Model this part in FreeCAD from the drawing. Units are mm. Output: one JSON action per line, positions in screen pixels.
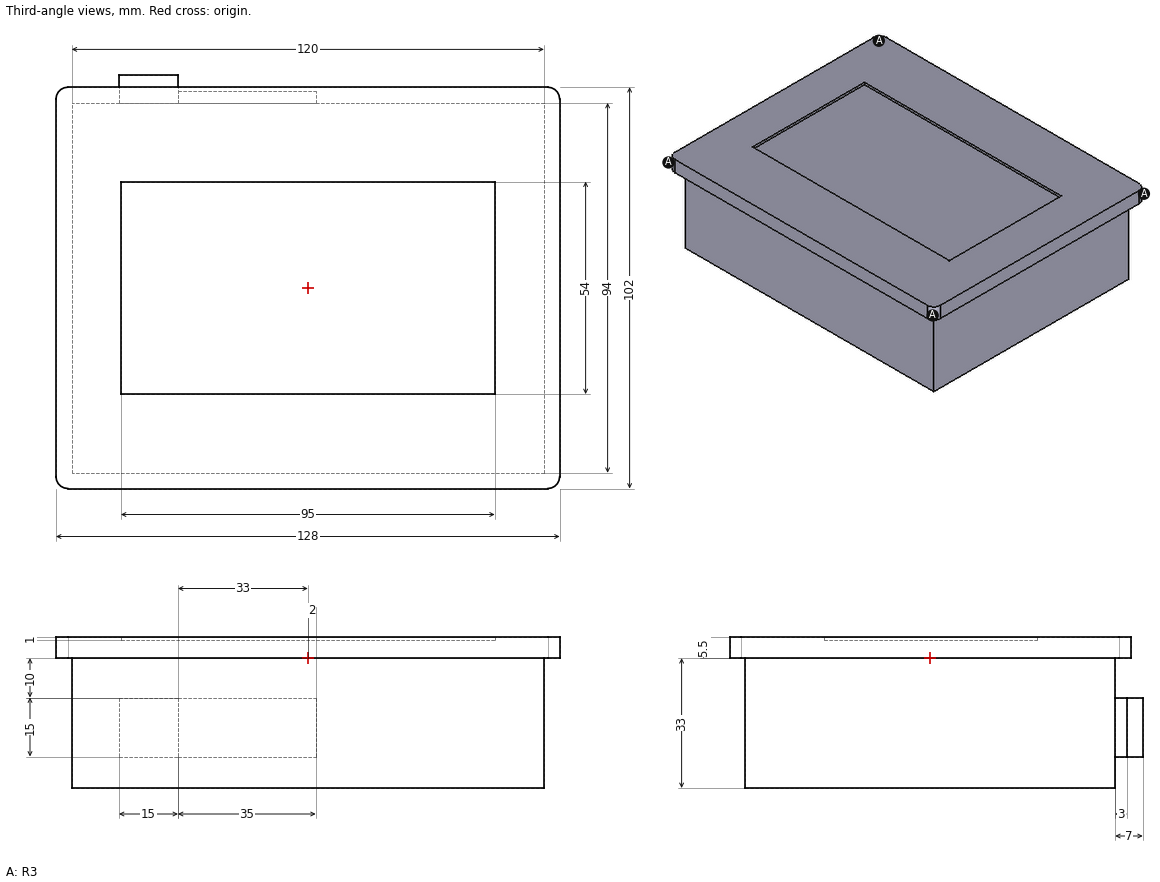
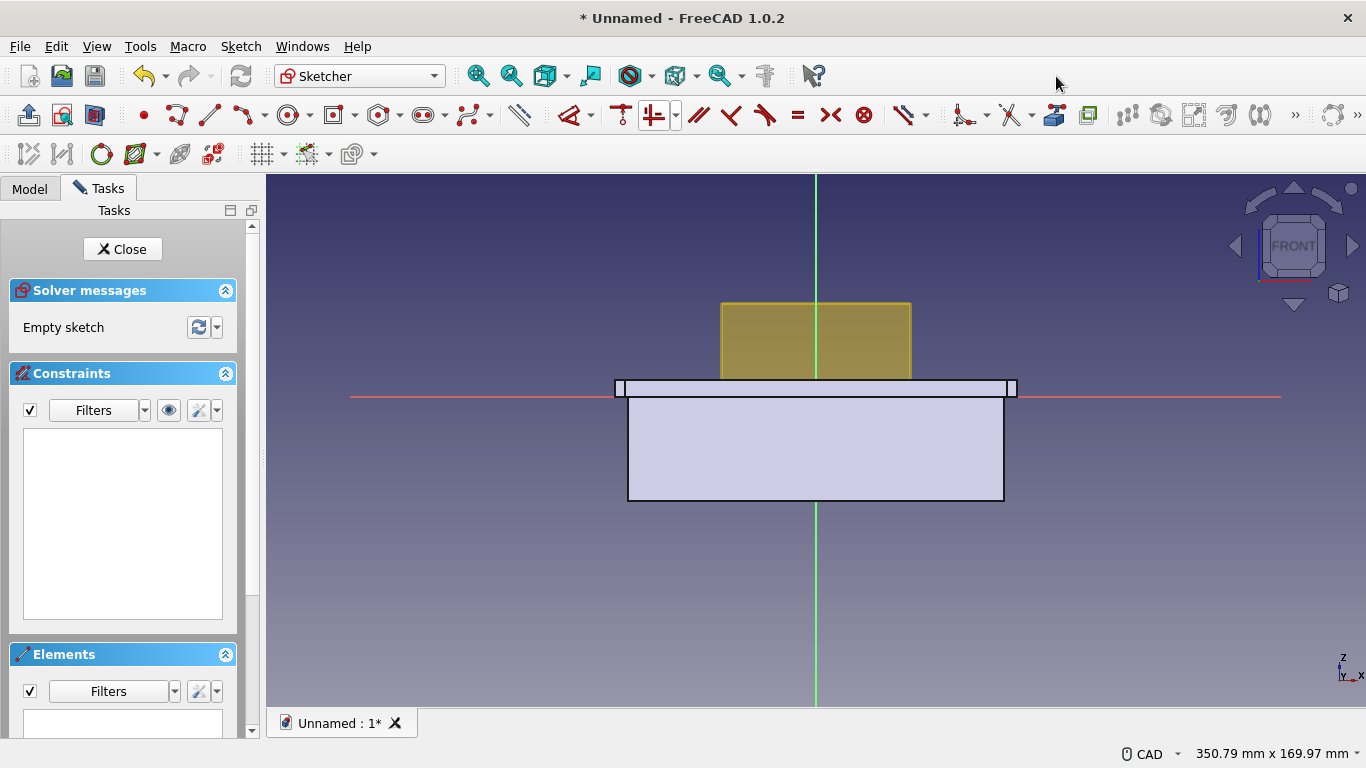
{"action": "scroll", "coordinate": [774, 435], "scroll_direction": "up", "scroll_amount": 7}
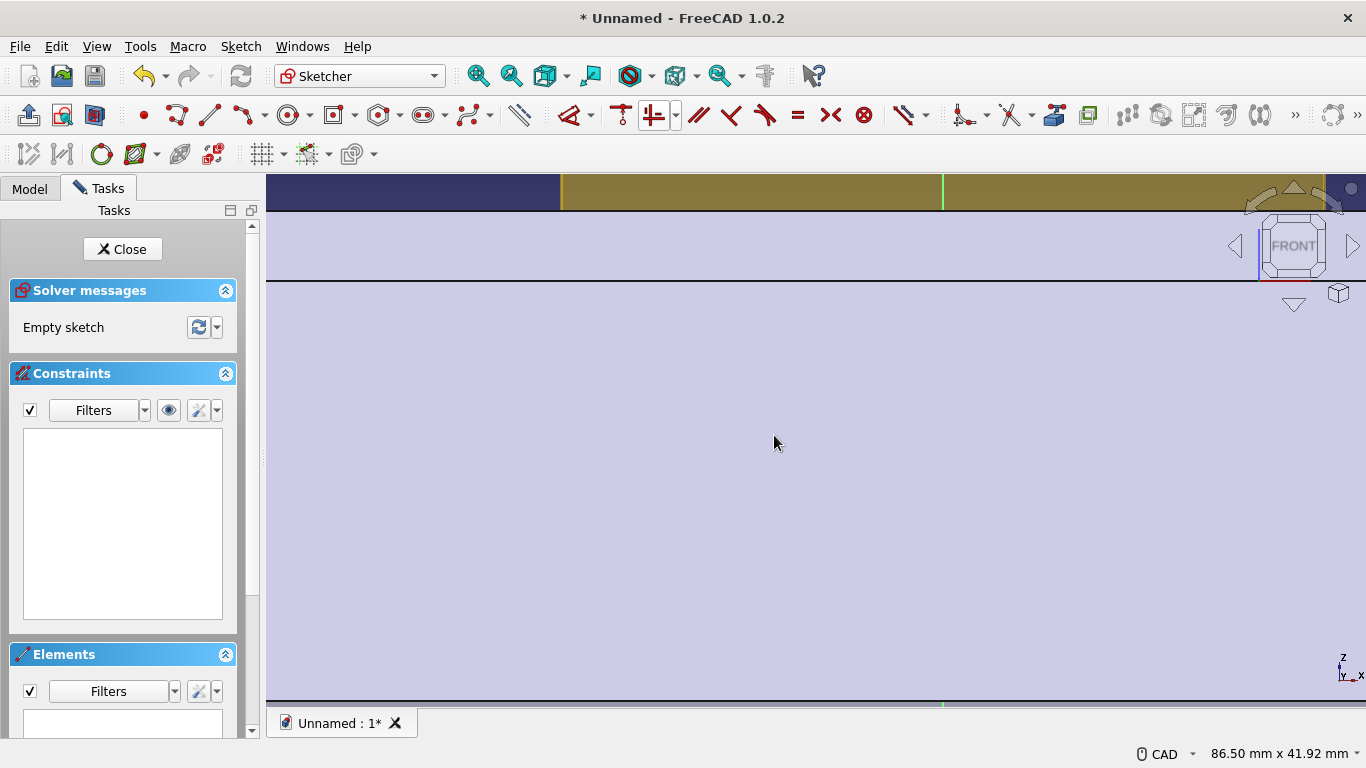
{"action": "key", "text": "g r"}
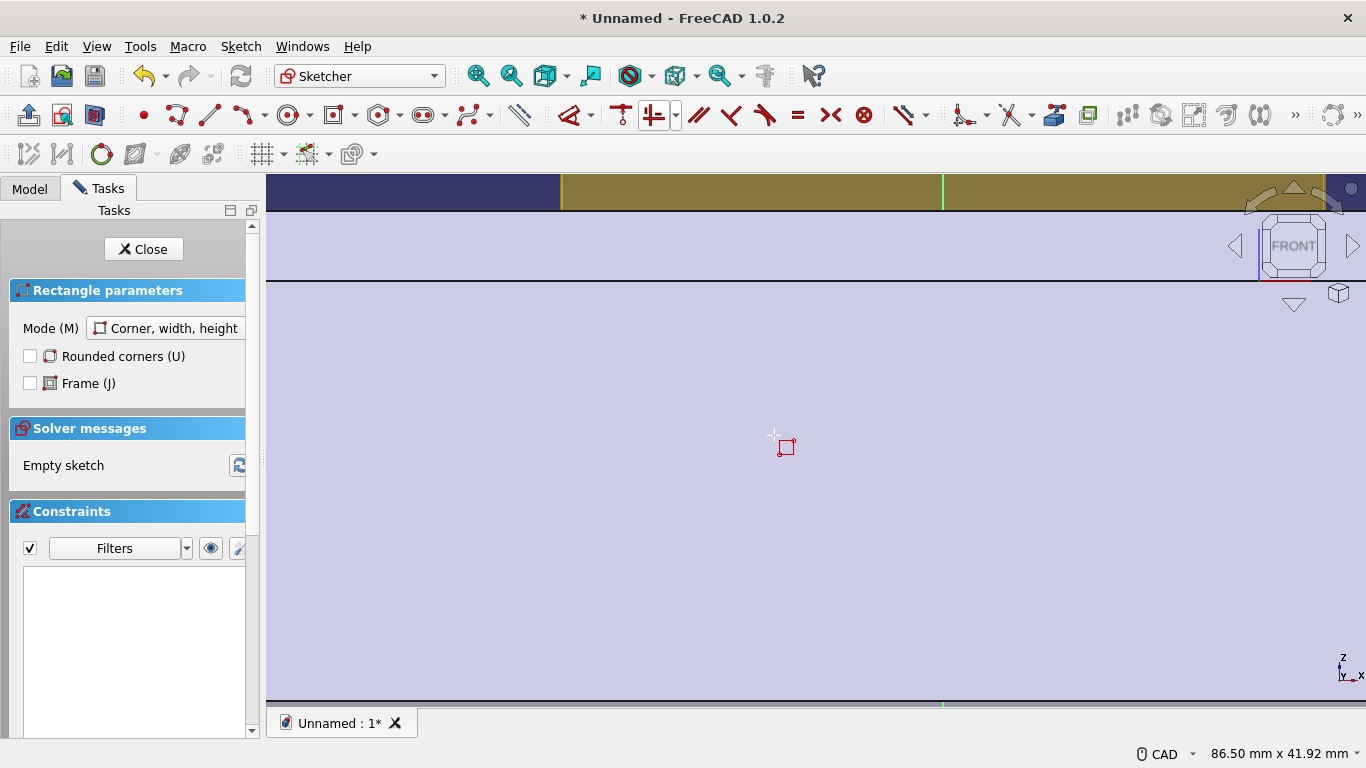
{"action": "left_click", "coordinate": [523, 408]}
{"action": "mouse_move", "coordinate": [968, 599]}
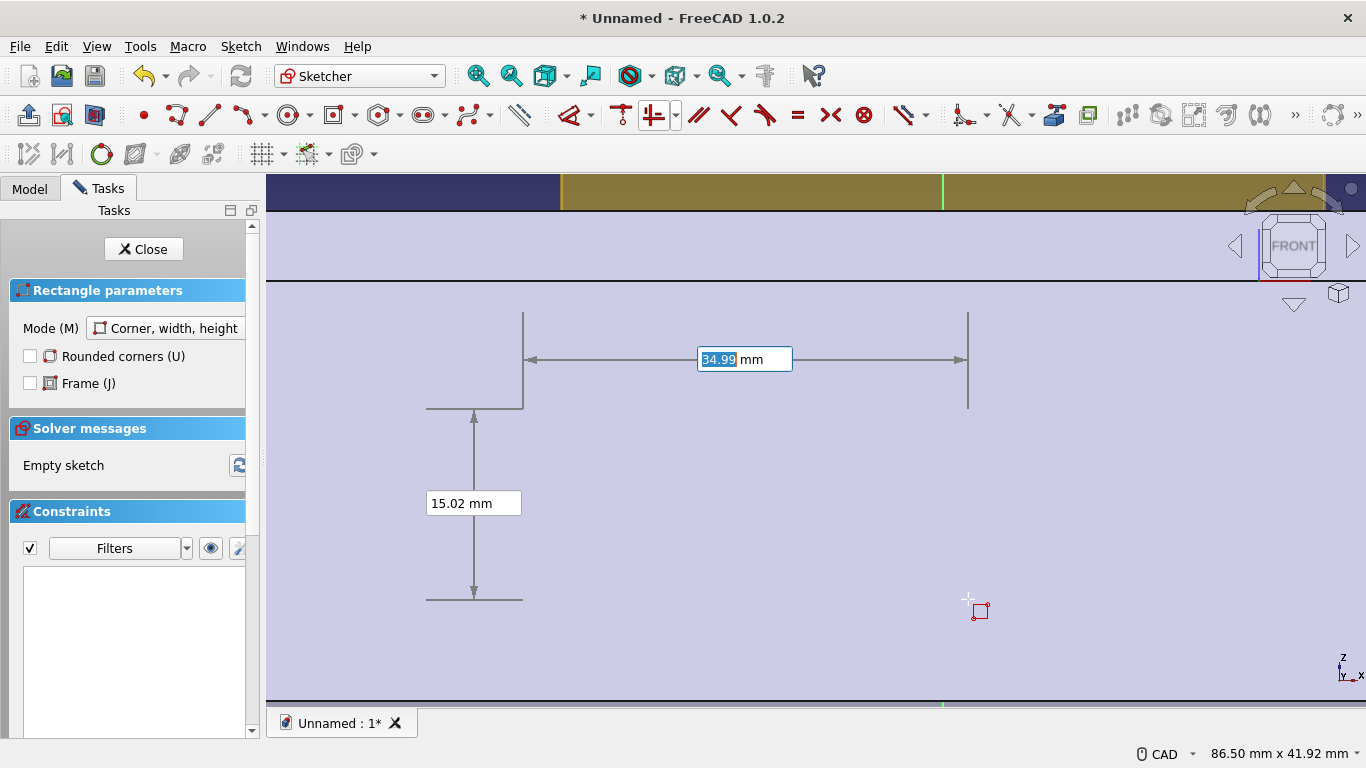
{"action": "type", "text": "35"}
{"action": "key", "text": "Tab"}
{"action": "type", "text": "15"}
{"action": "key", "text": "Return"}
{"action": "key", "text": "Escape"}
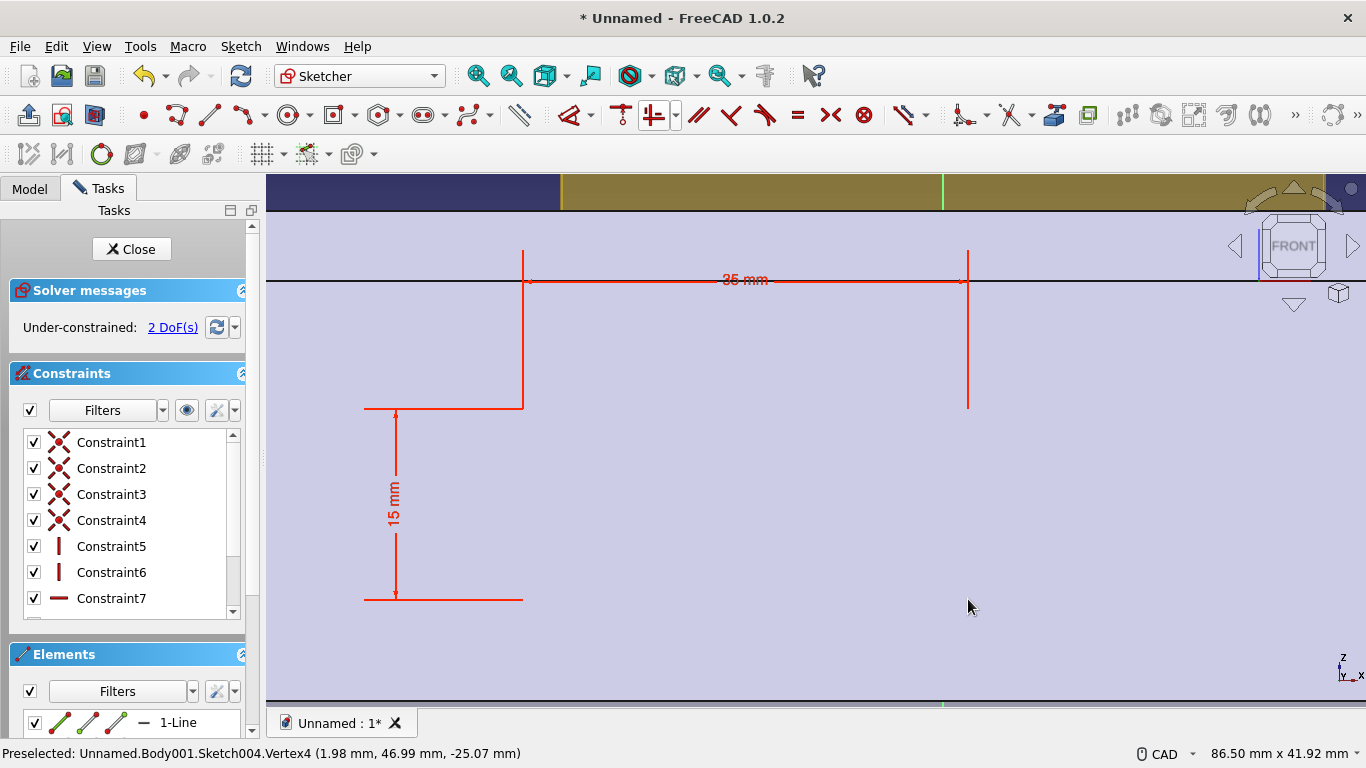
{"action": "left_click", "coordinate": [568, 116]}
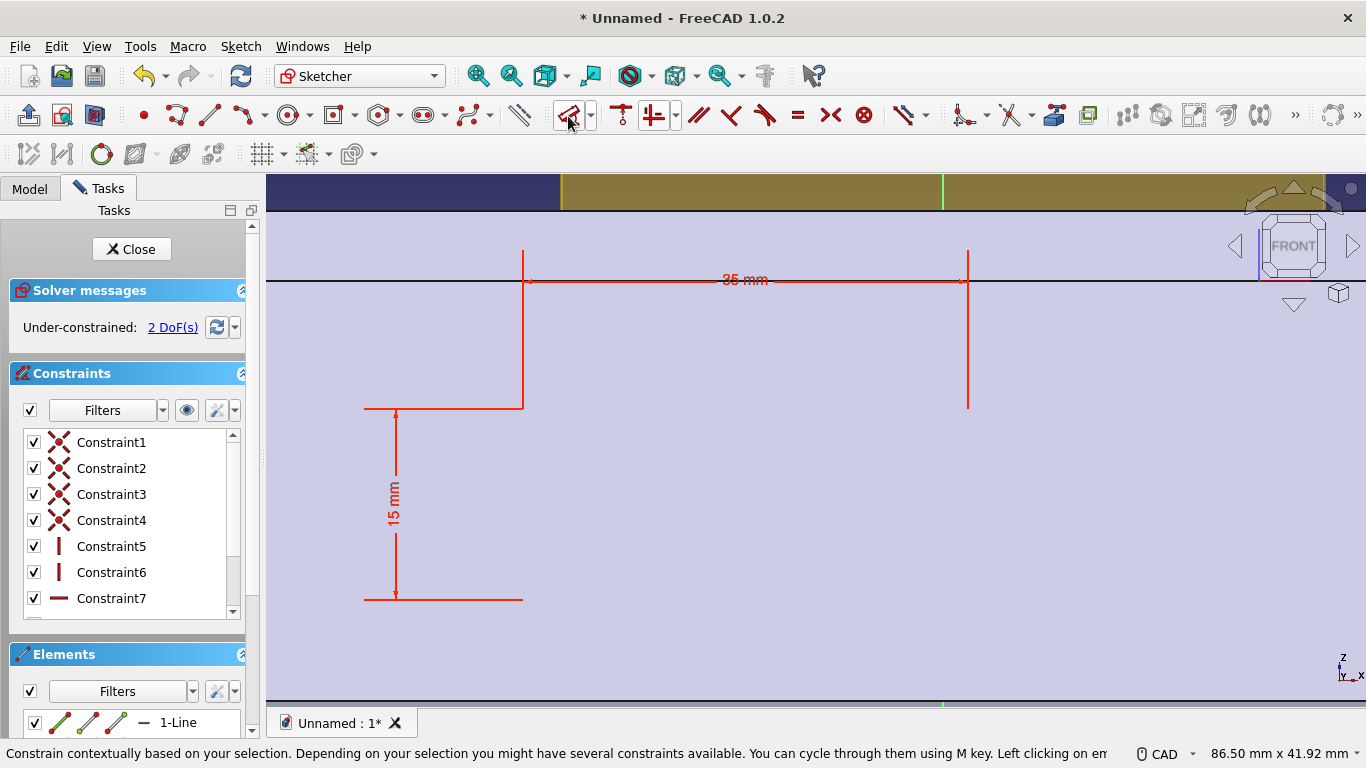
{"action": "scroll", "coordinate": [968, 600], "scroll_direction": "up", "scroll_amount": 3}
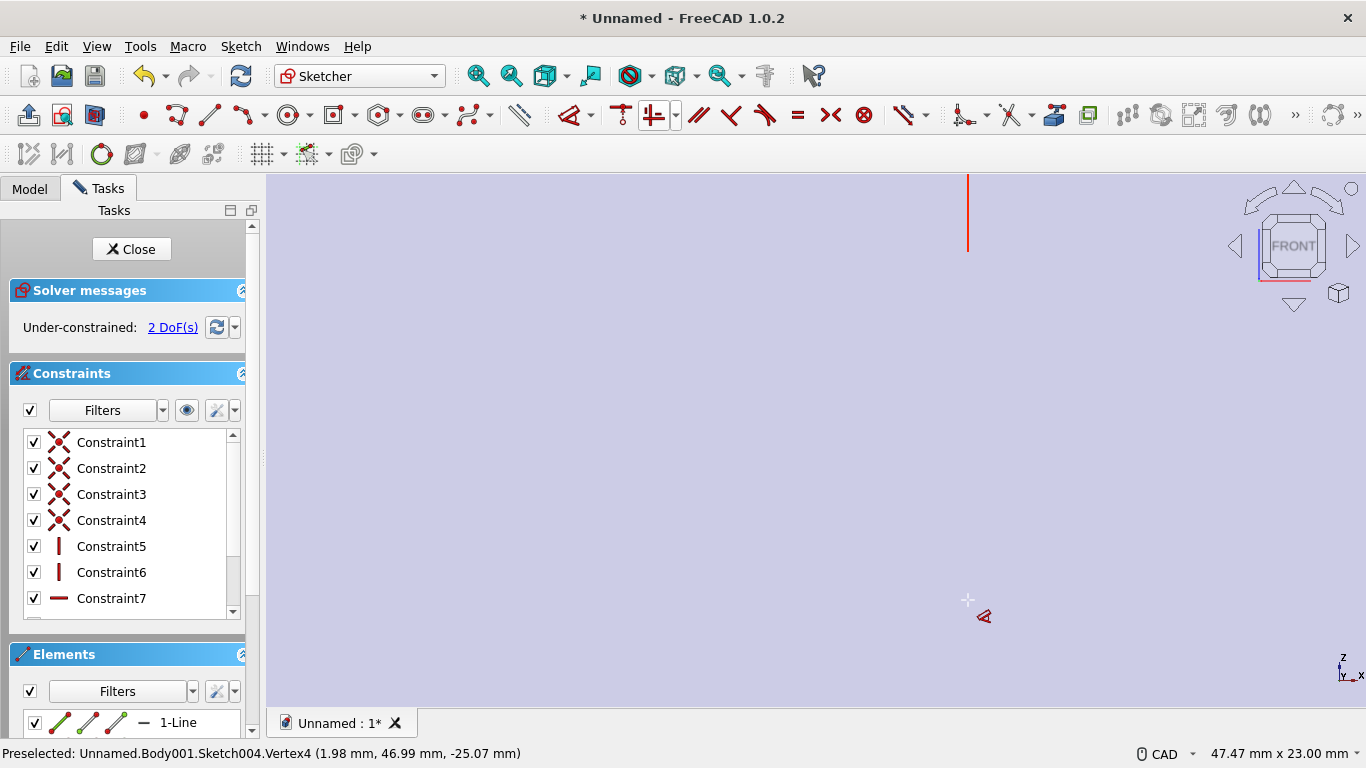
{"action": "left_click", "coordinate": [968, 599]}
{"action": "left_click", "coordinate": [945, 633]}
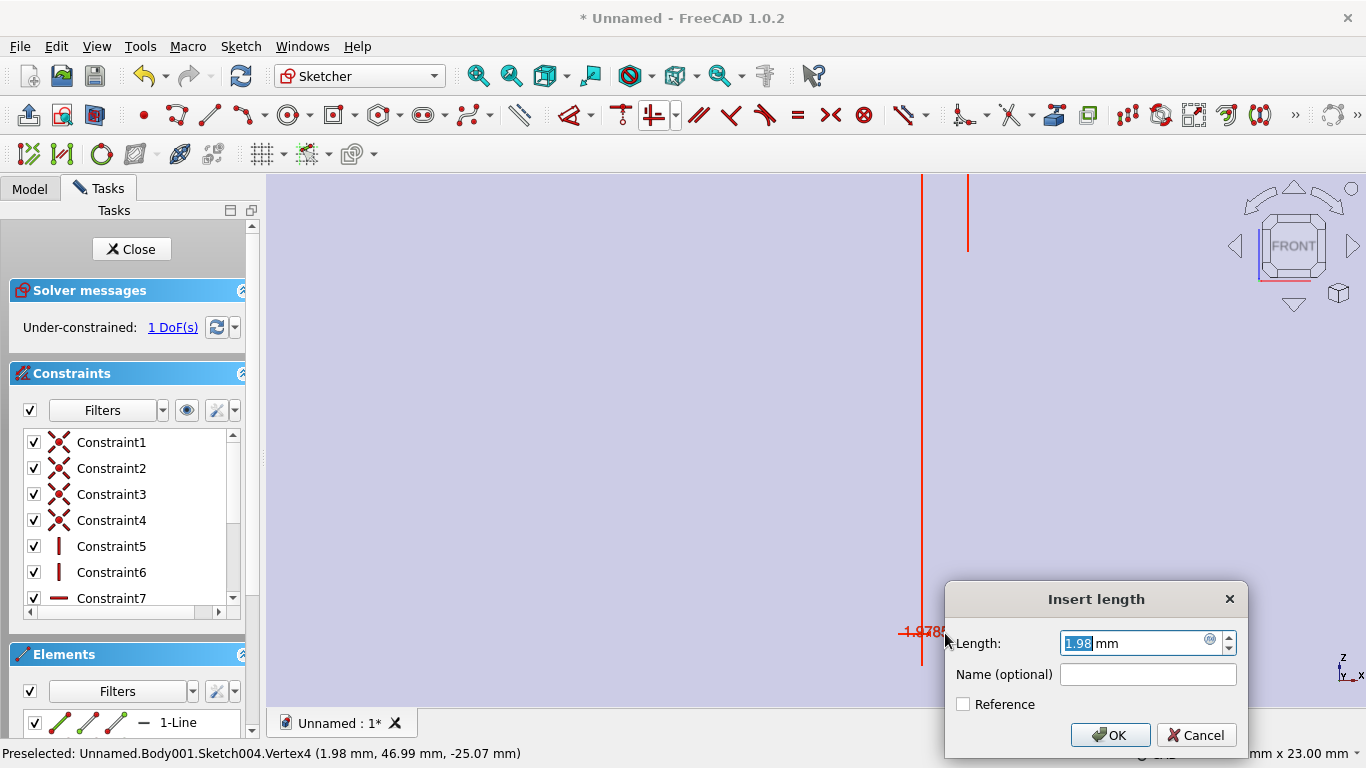
{"action": "type", "text": "2"}
{"action": "key", "text": "Return"}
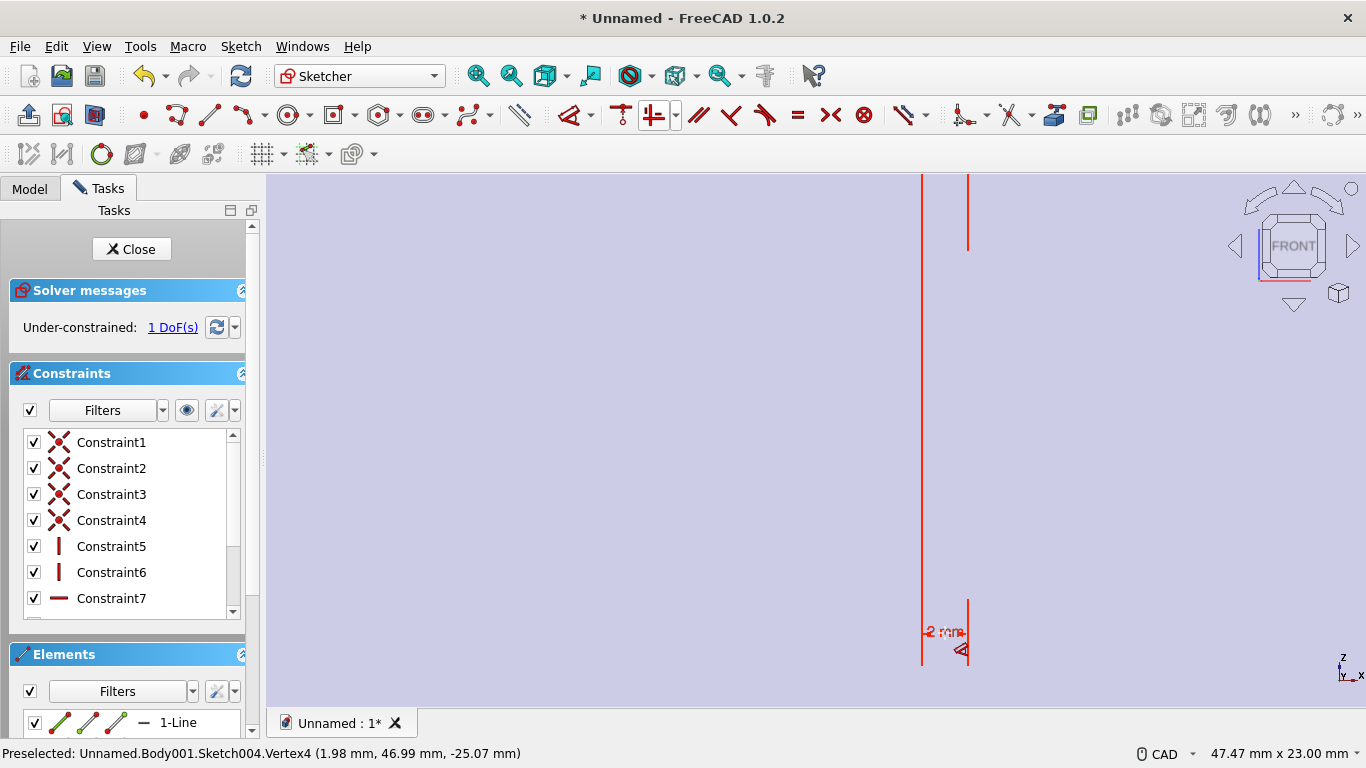
{"action": "scroll", "coordinate": [972, 602], "scroll_direction": "down", "scroll_amount": 3}